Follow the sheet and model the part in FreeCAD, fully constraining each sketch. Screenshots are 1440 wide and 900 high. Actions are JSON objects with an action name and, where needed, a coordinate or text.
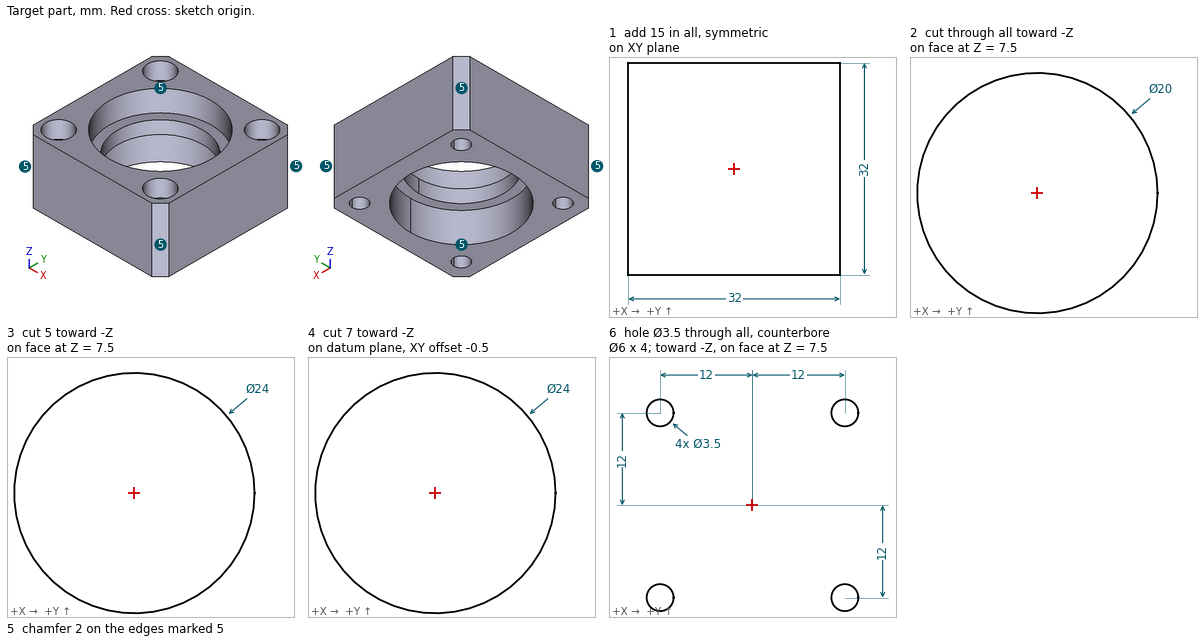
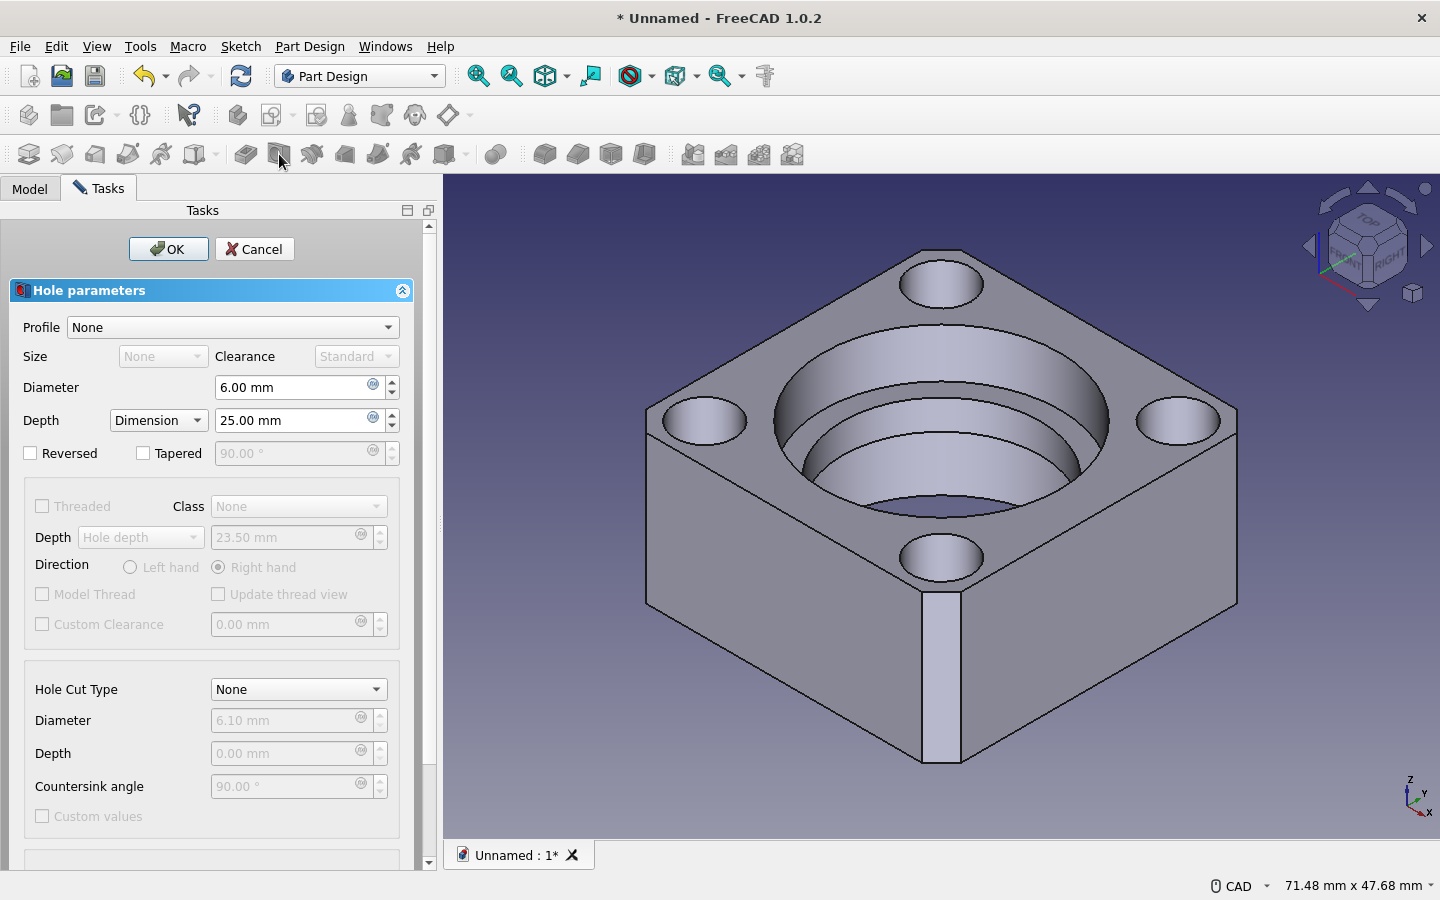
{"action": "triple_click", "coordinate": [300, 388]}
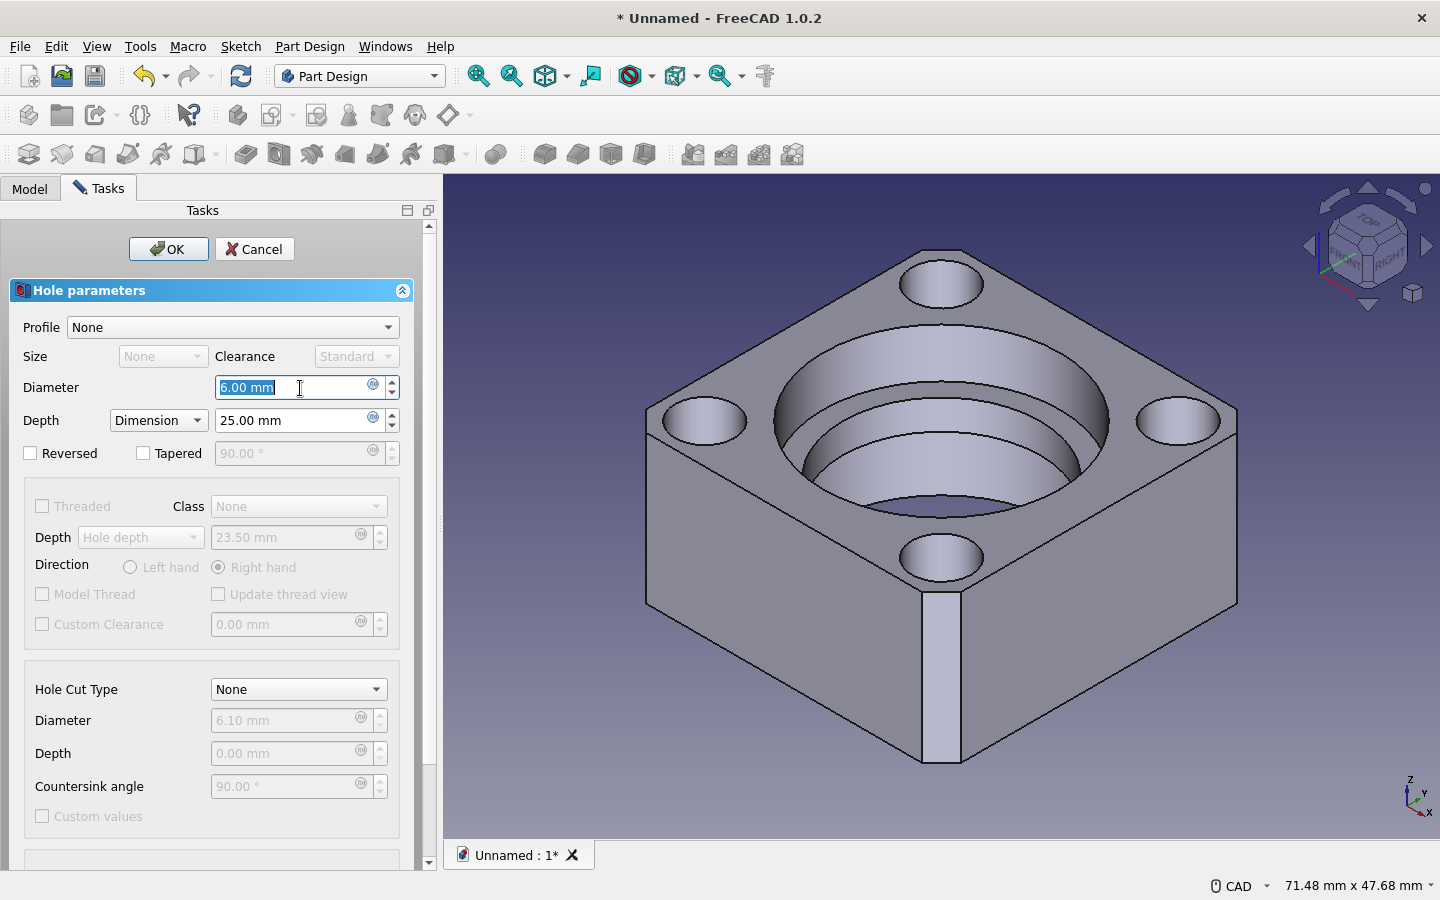
{"action": "type", "text": "3.5"}
{"action": "key", "text": "Tab"}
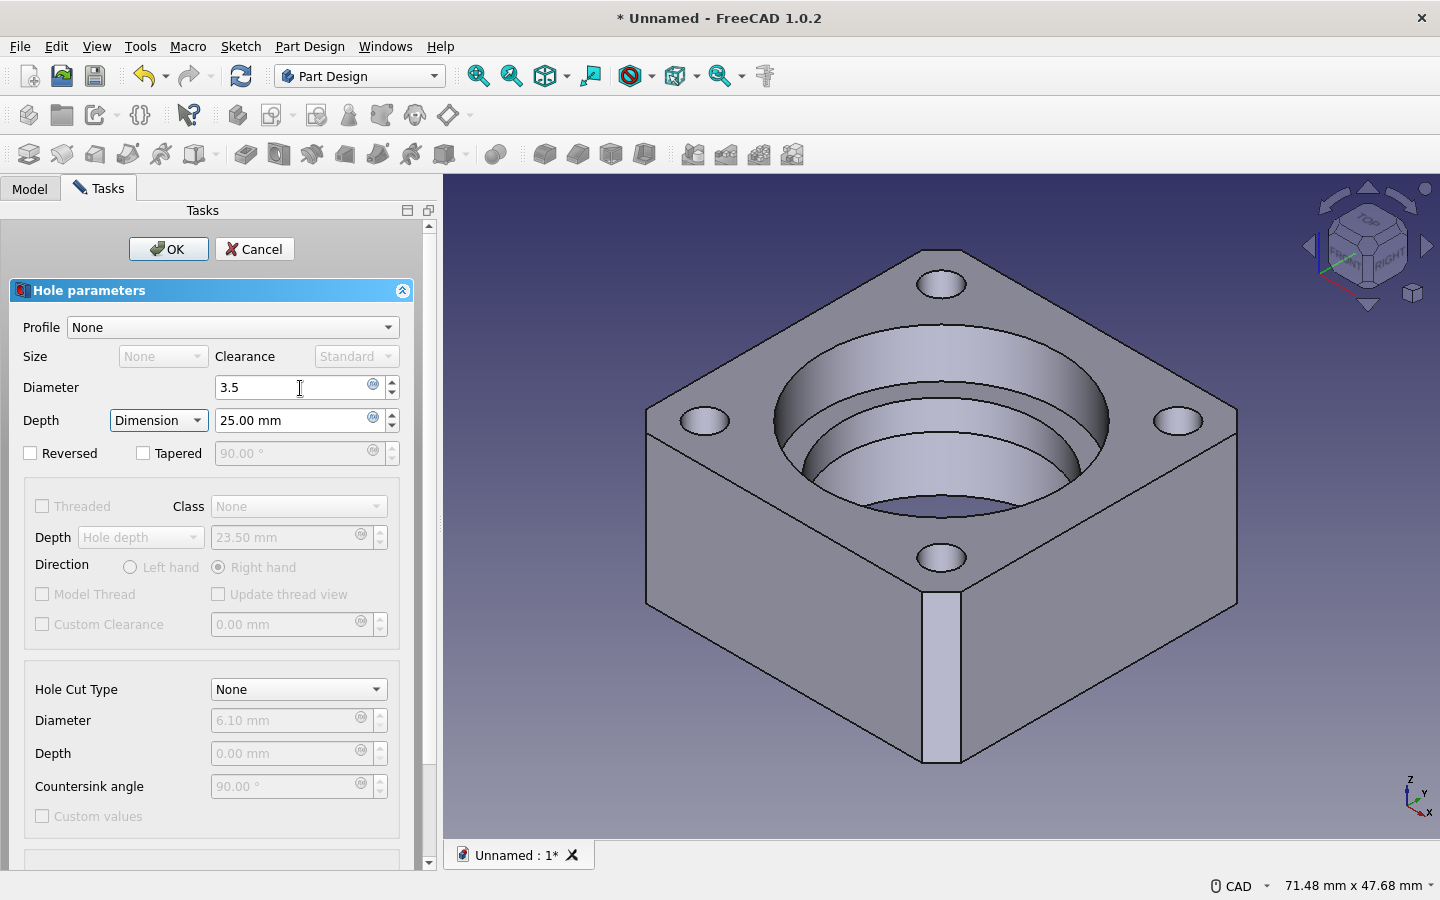
{"action": "left_click", "coordinate": [160, 420]}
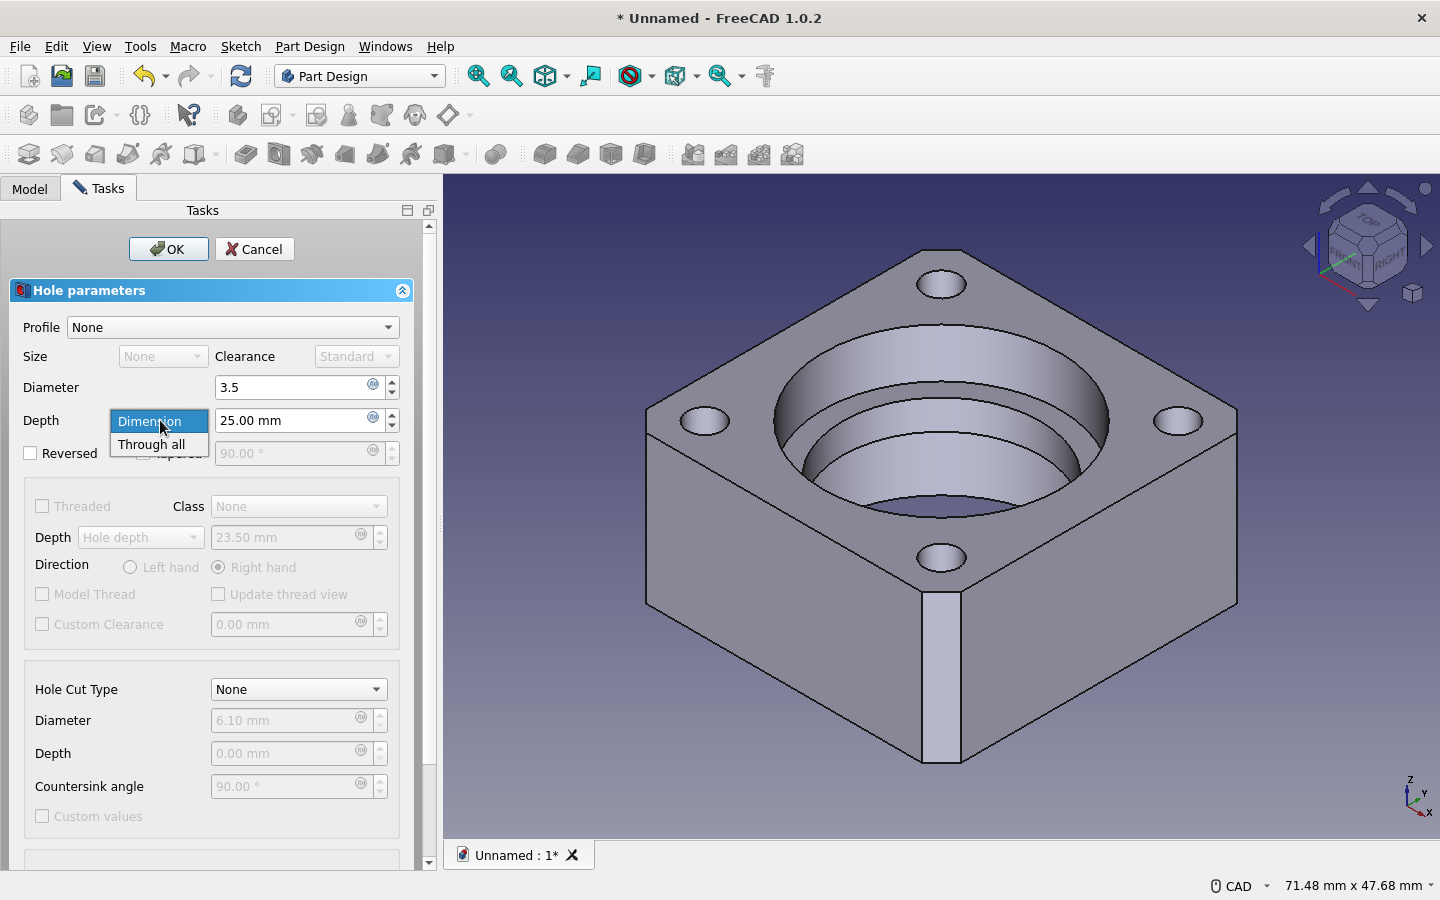
{"action": "left_click", "coordinate": [158, 444]}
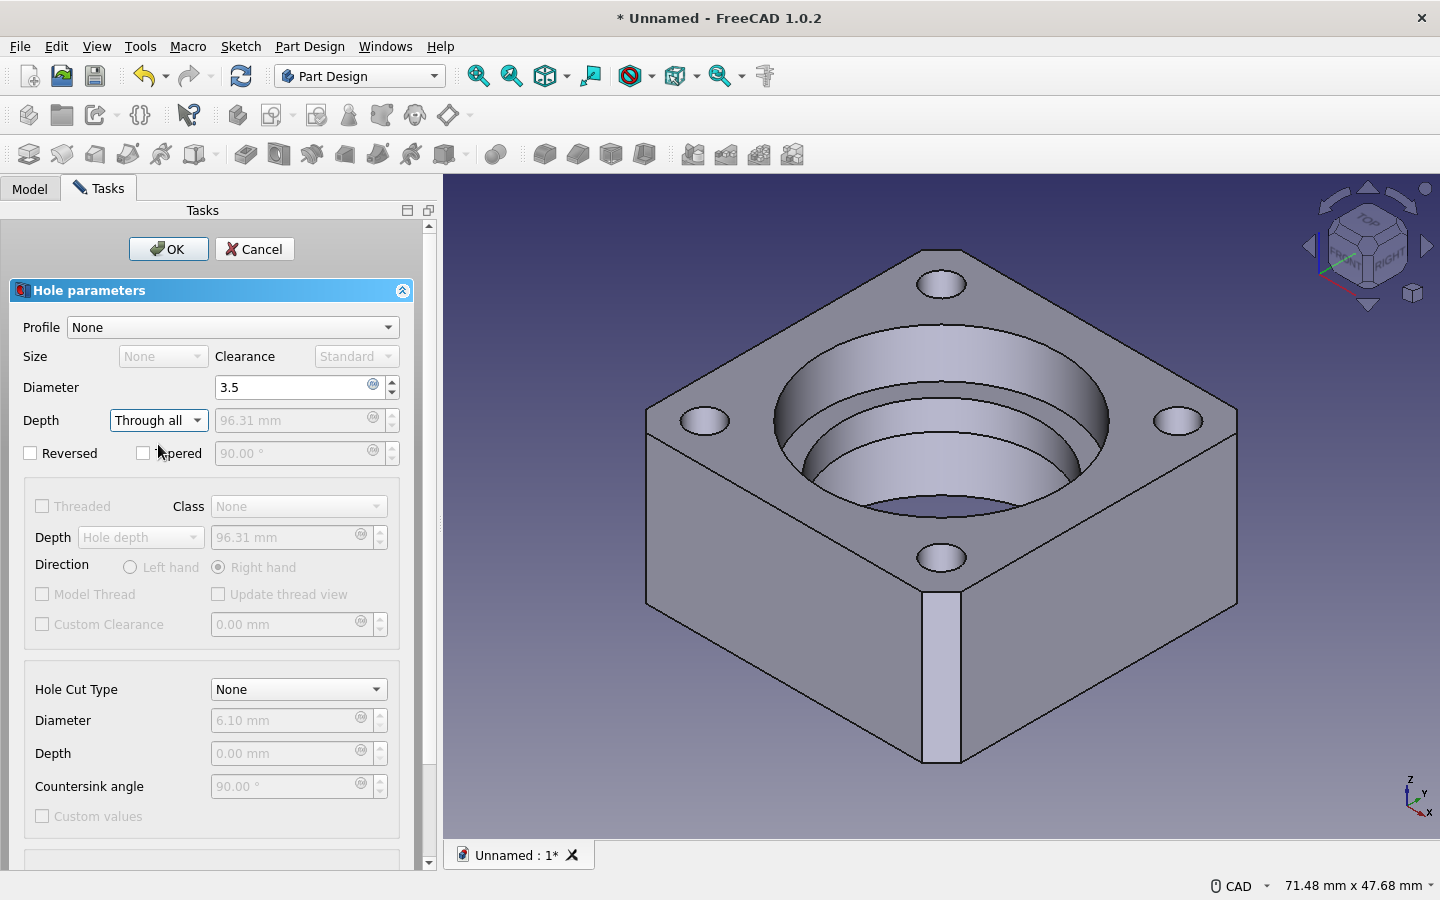
{"action": "left_click", "coordinate": [300, 690]}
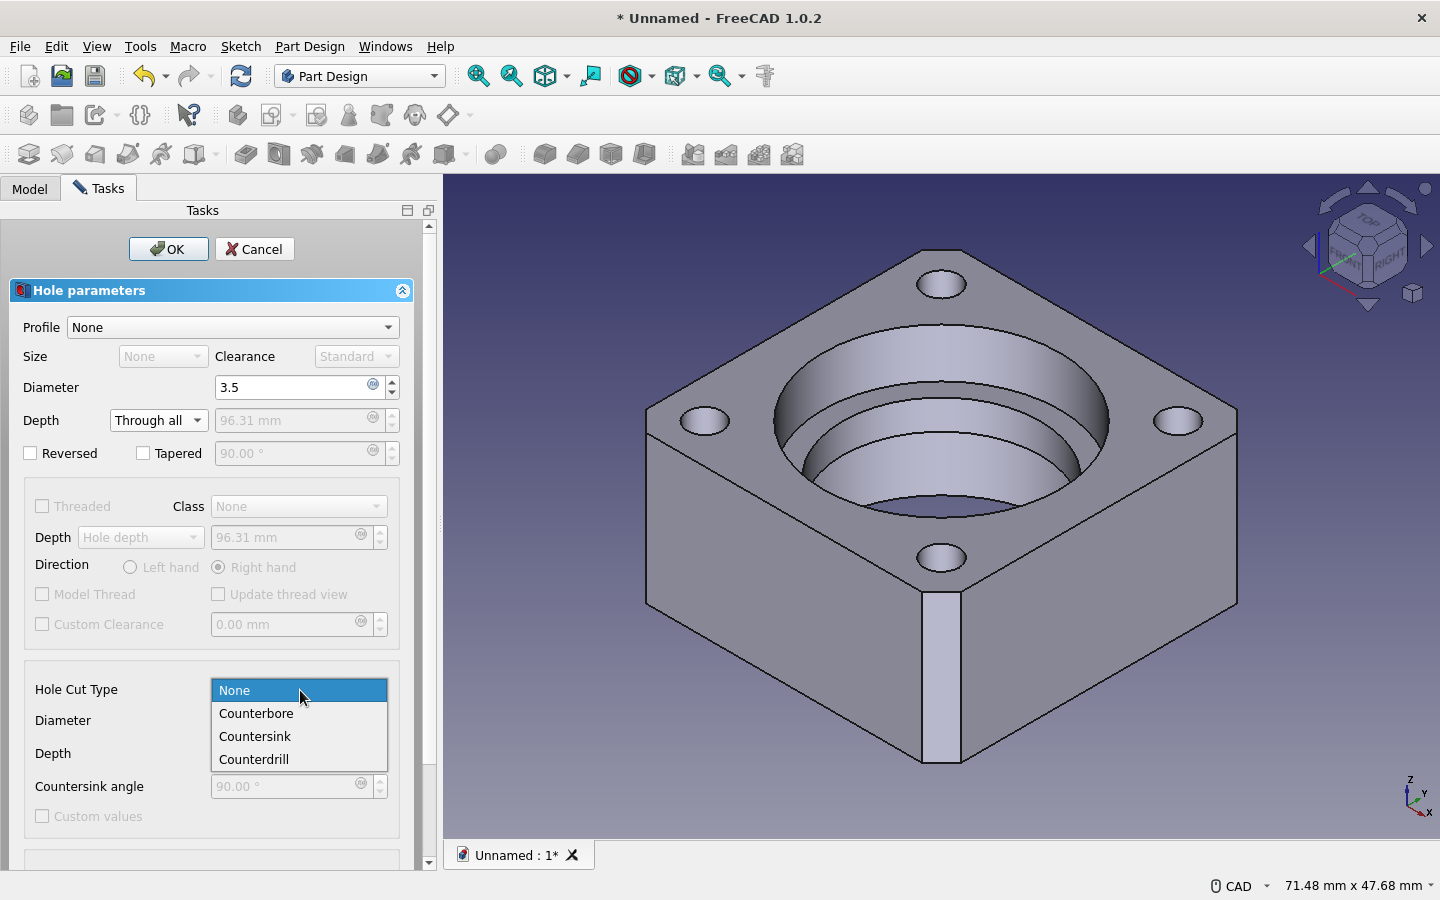
{"action": "left_click", "coordinate": [298, 714]}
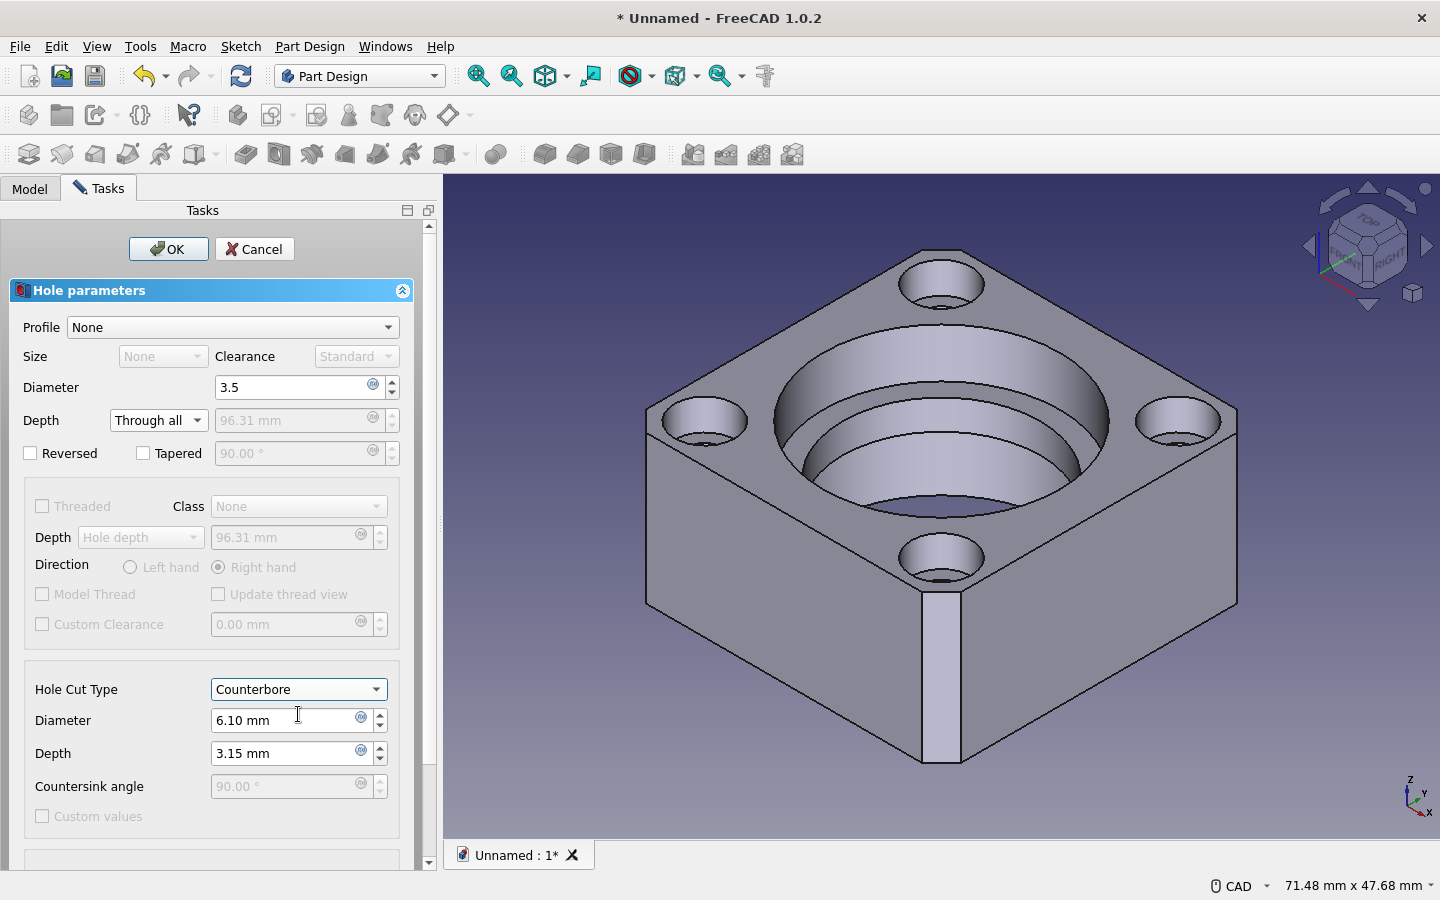
{"action": "triple_click", "coordinate": [292, 720]}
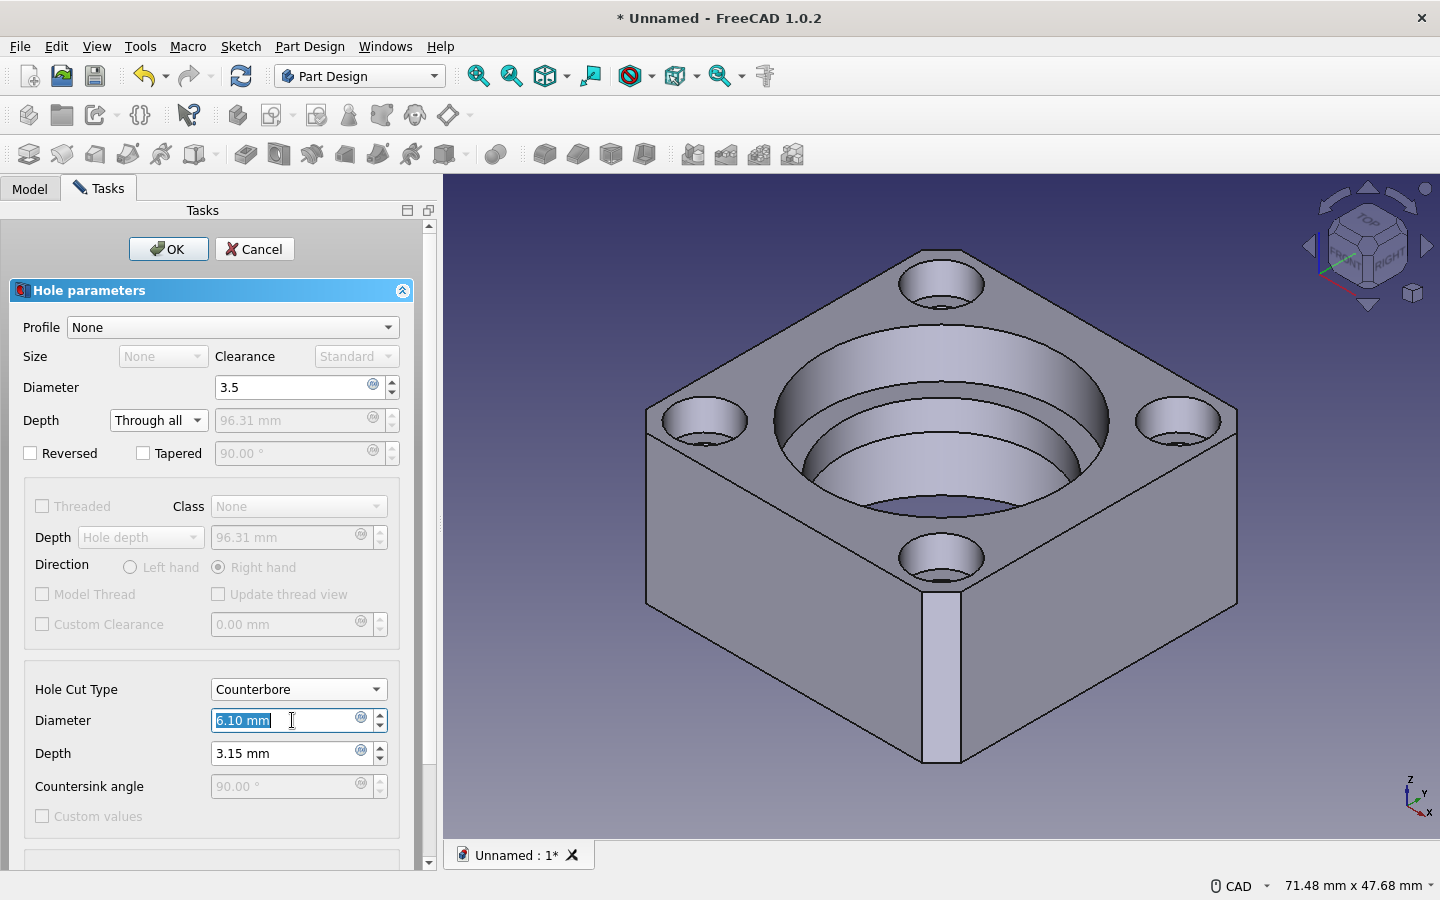
{"action": "type", "text": "6"}
{"action": "key", "text": "Tab"}